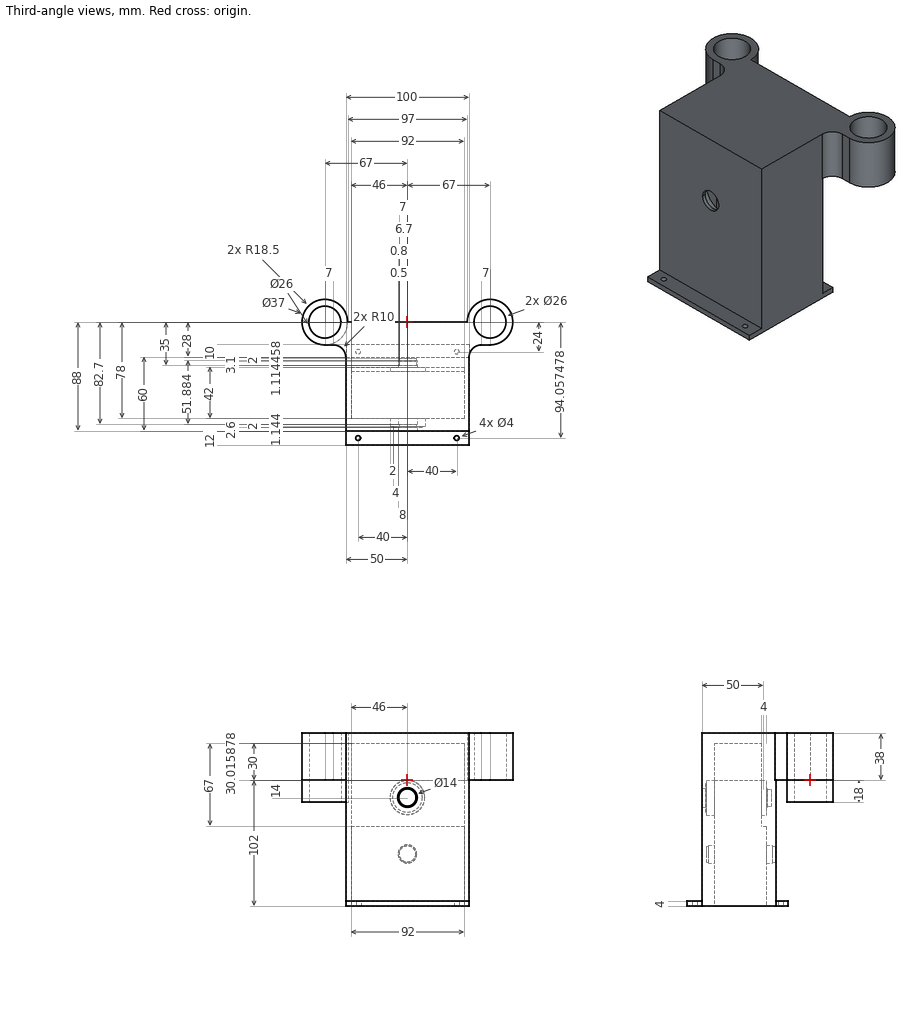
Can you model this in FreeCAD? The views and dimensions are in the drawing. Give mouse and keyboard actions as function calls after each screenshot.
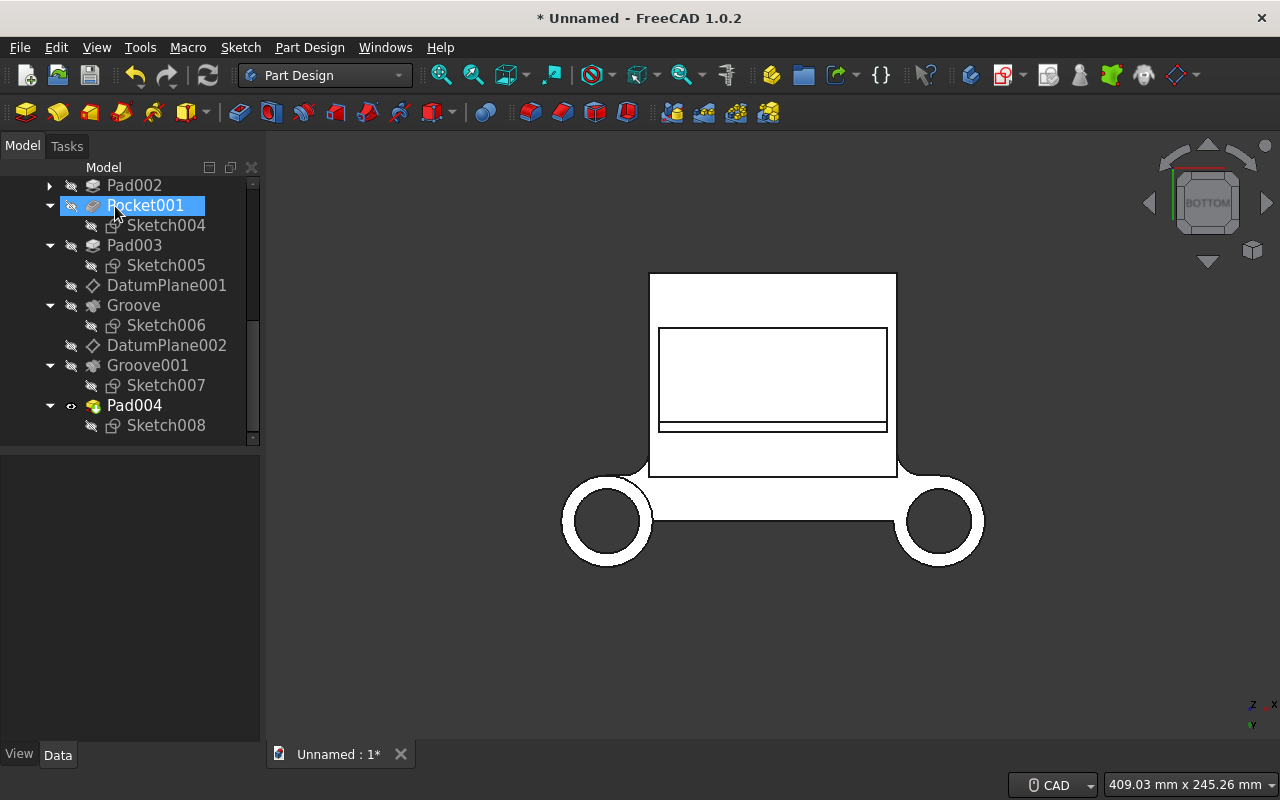
click(879, 461)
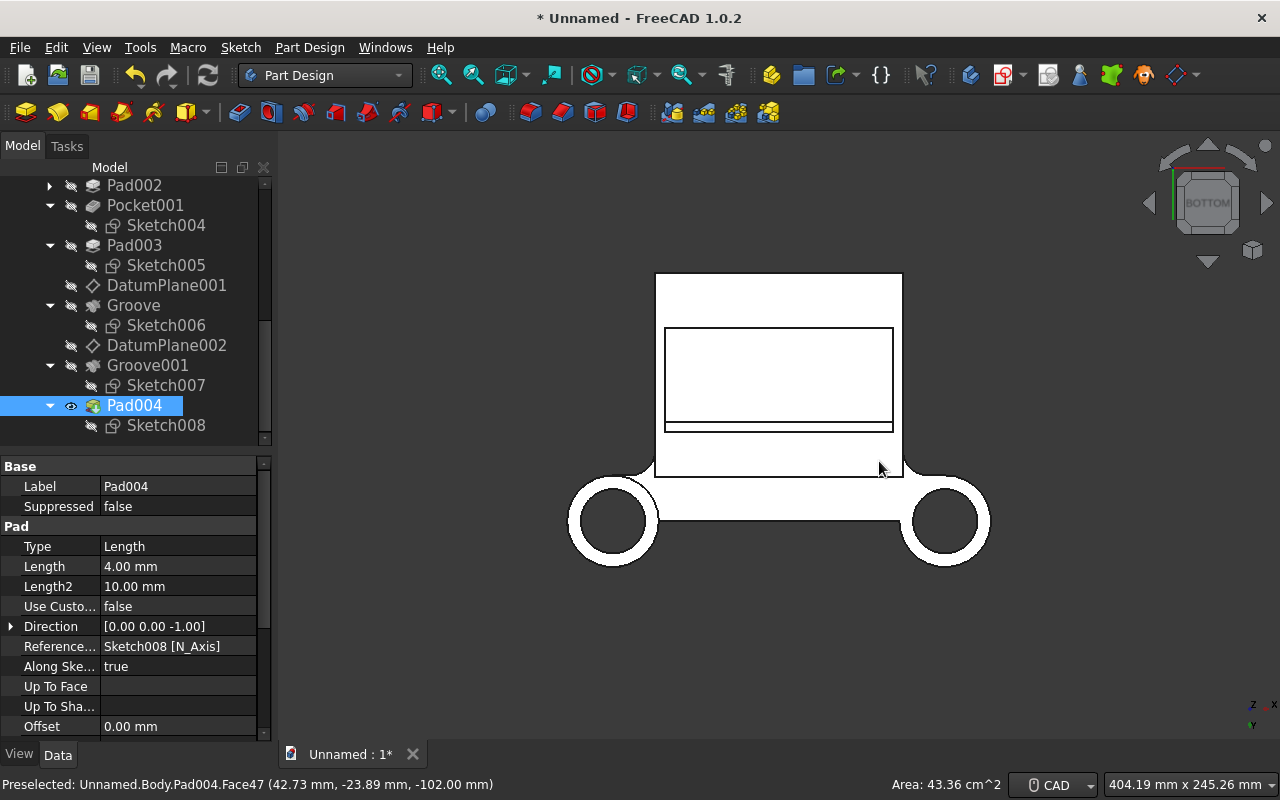
click(1004, 76)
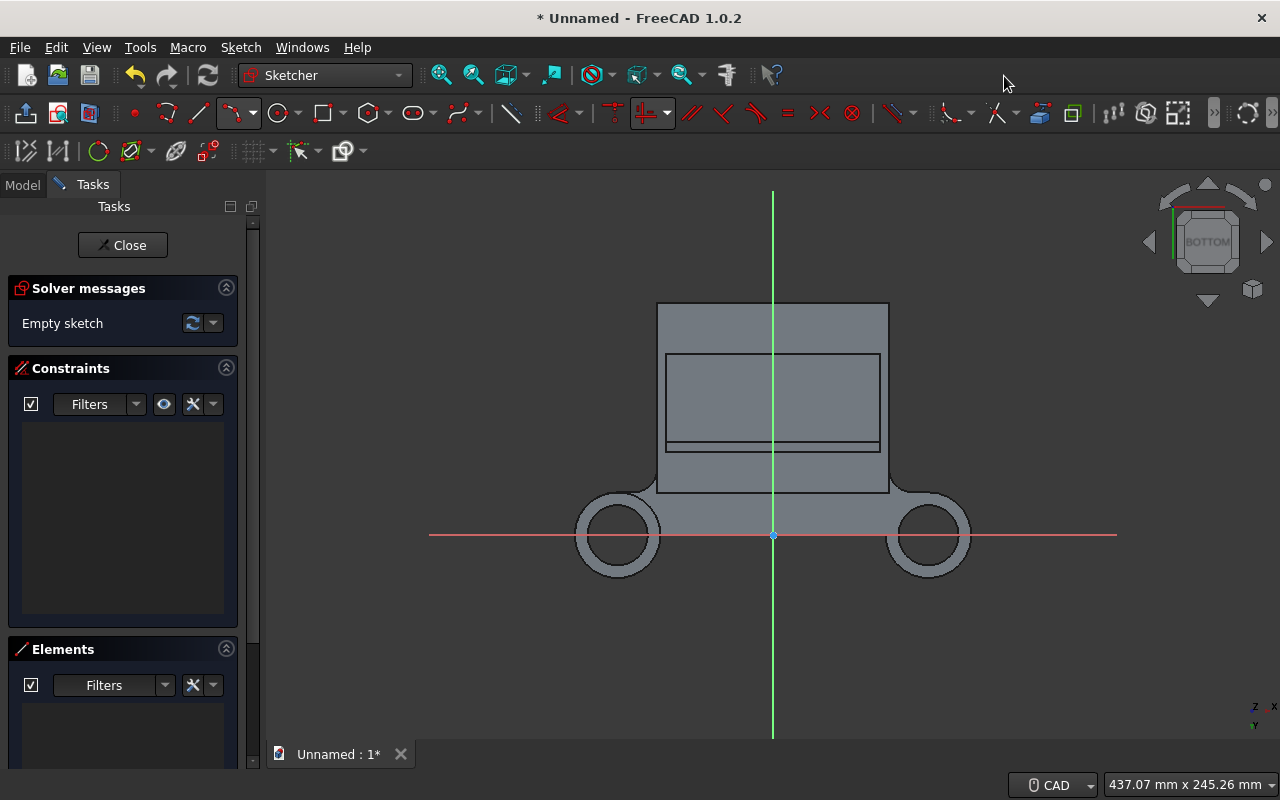
scroll(912, 361, up, 2)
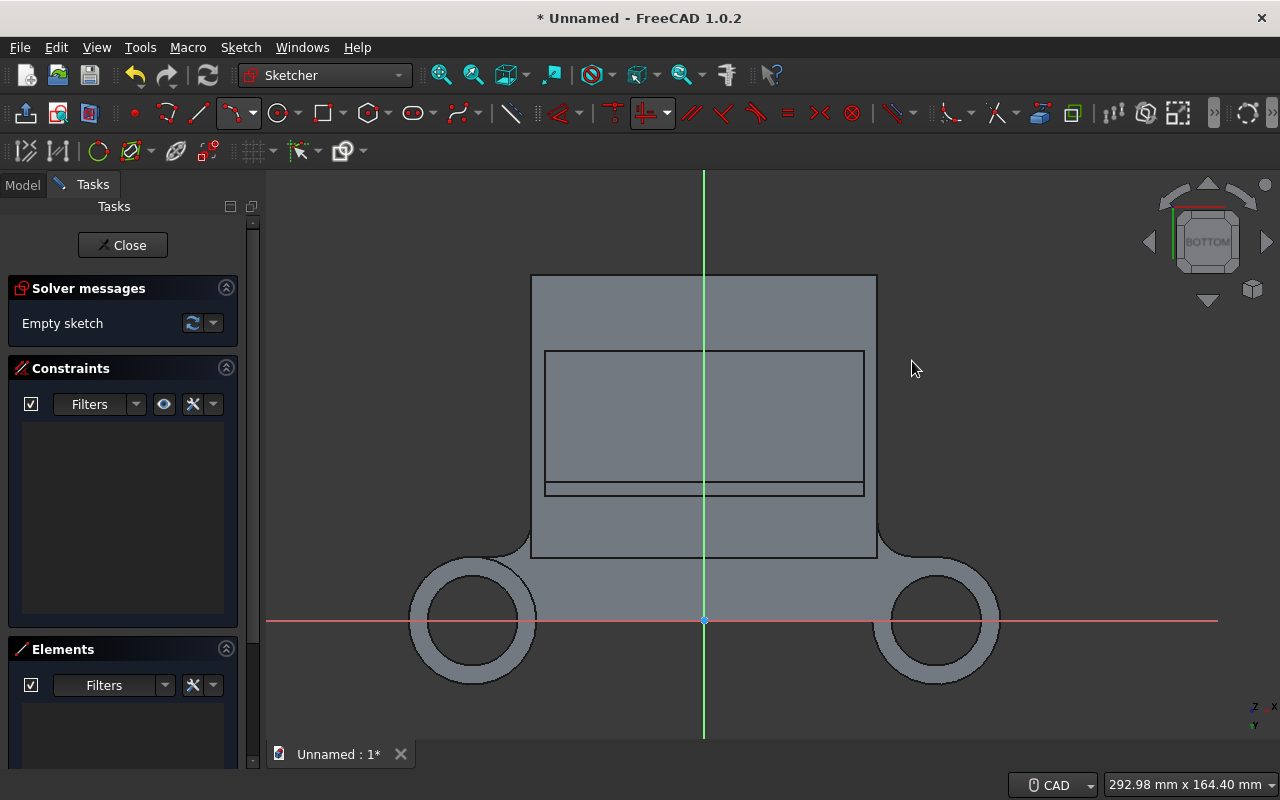
key(g)
key(c)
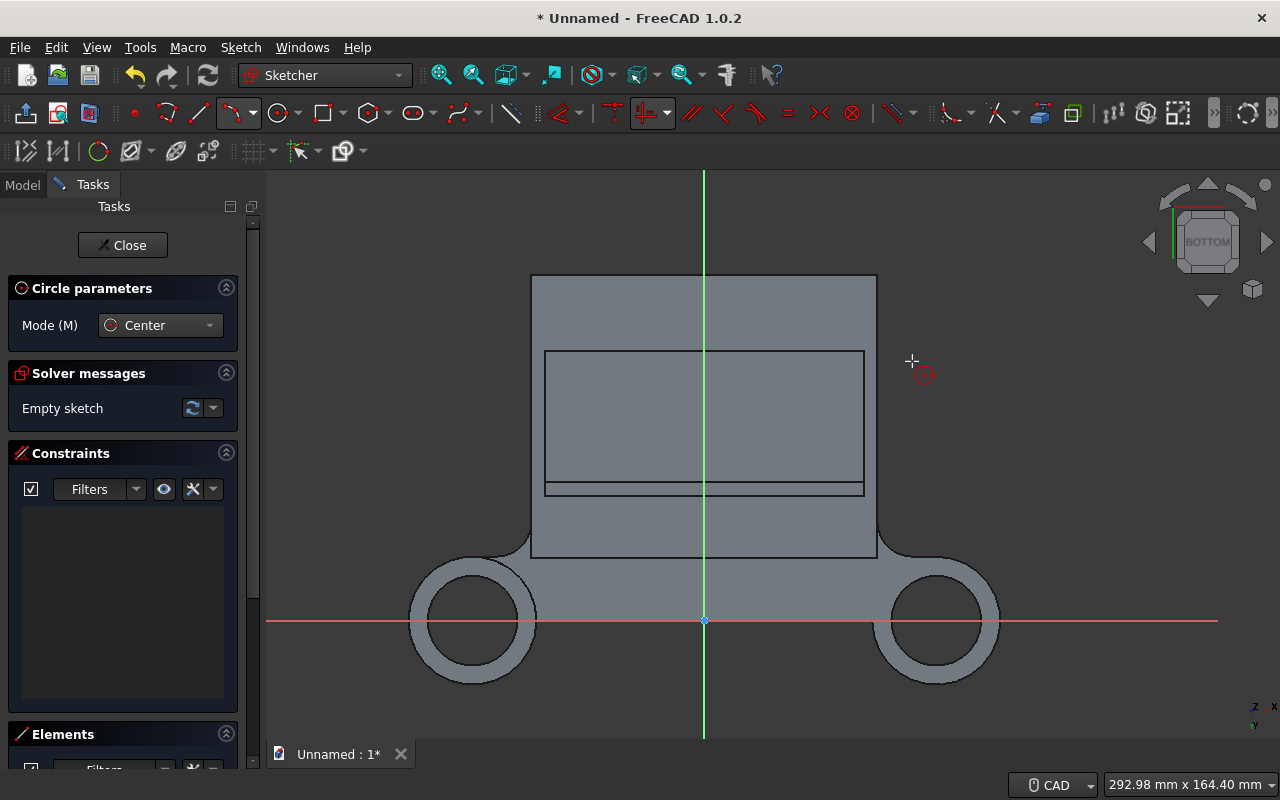
scroll(843, 295, up, 6)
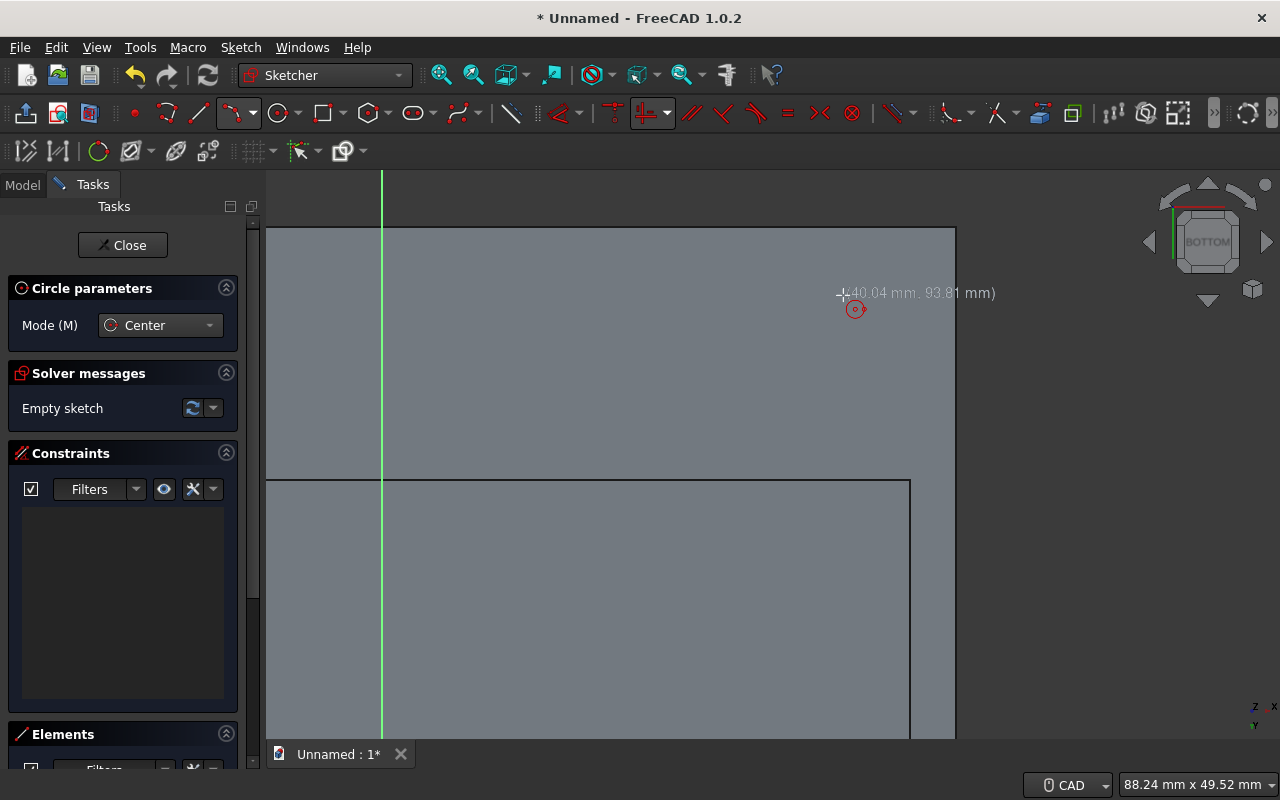
click(841, 295)
click(857, 279)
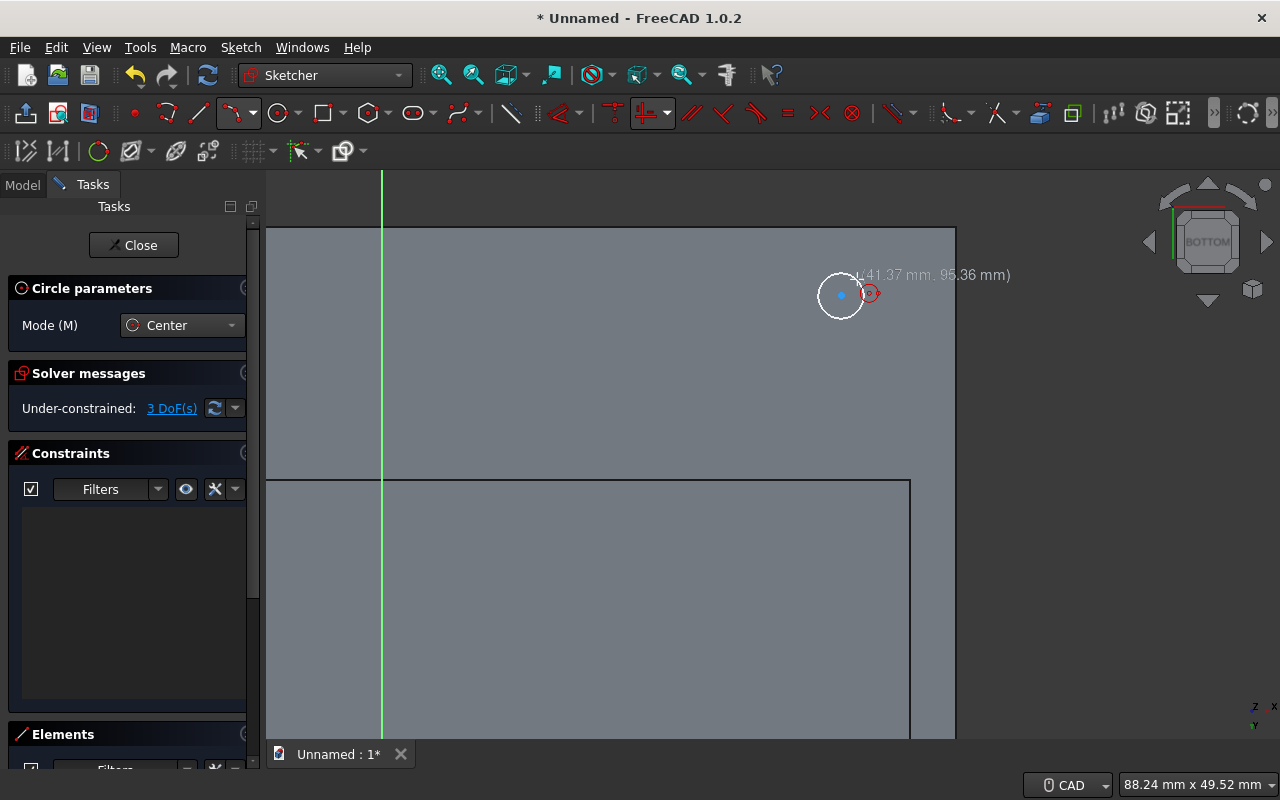
scroll(844, 295, down, 6)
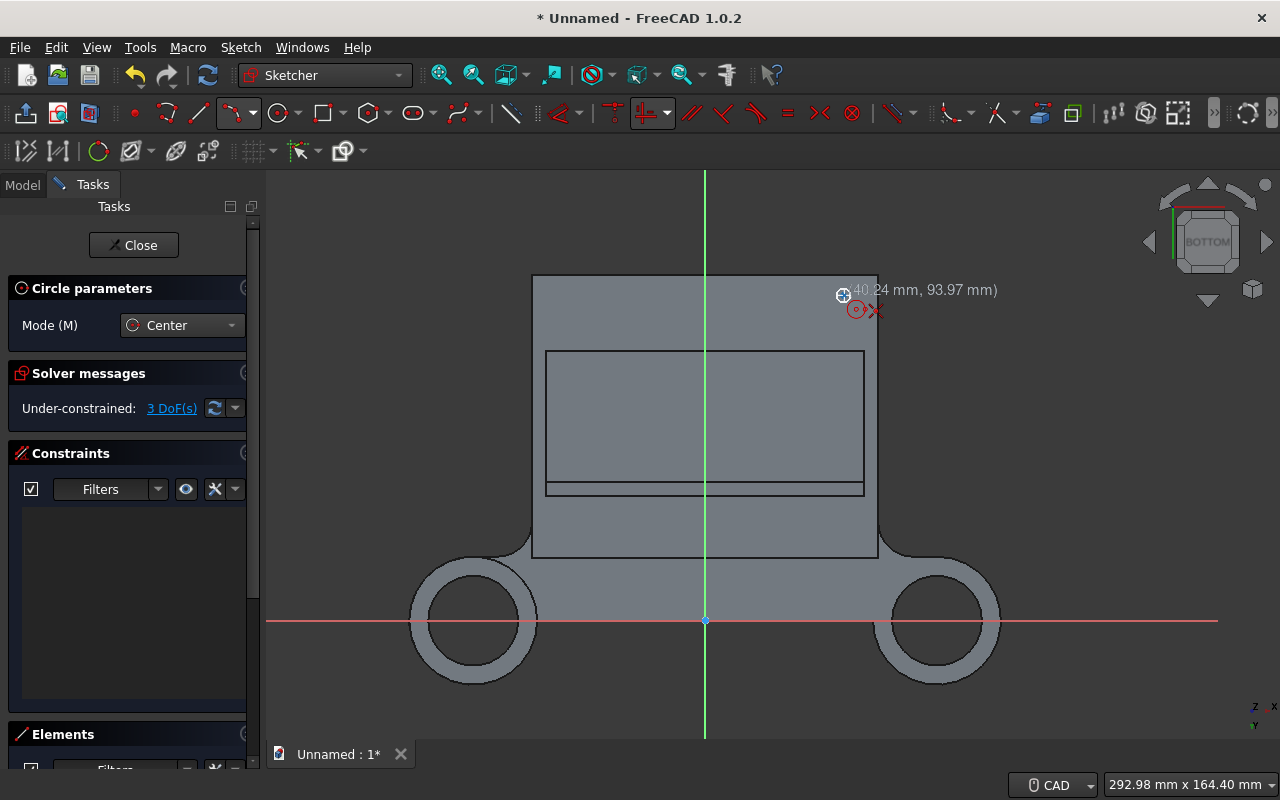
scroll(844, 538, up, 6)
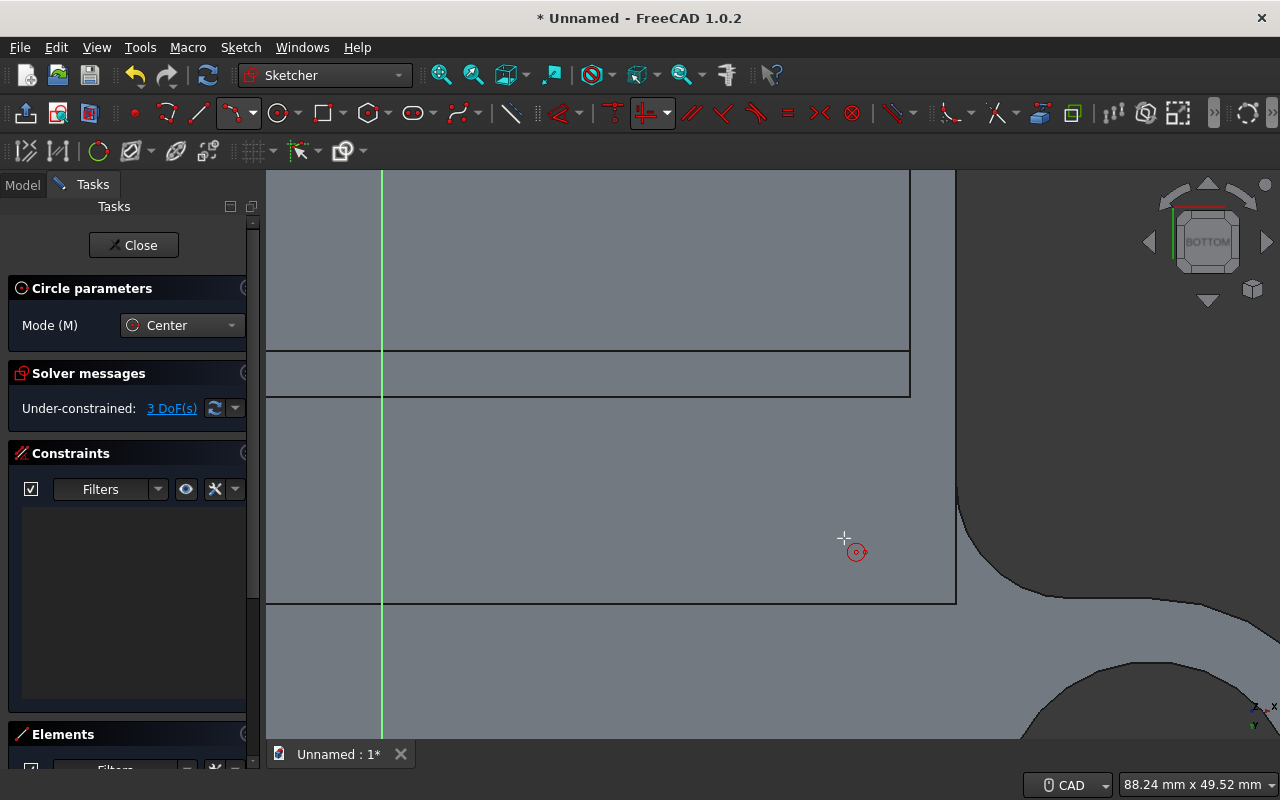
click(841, 535)
click(857, 519)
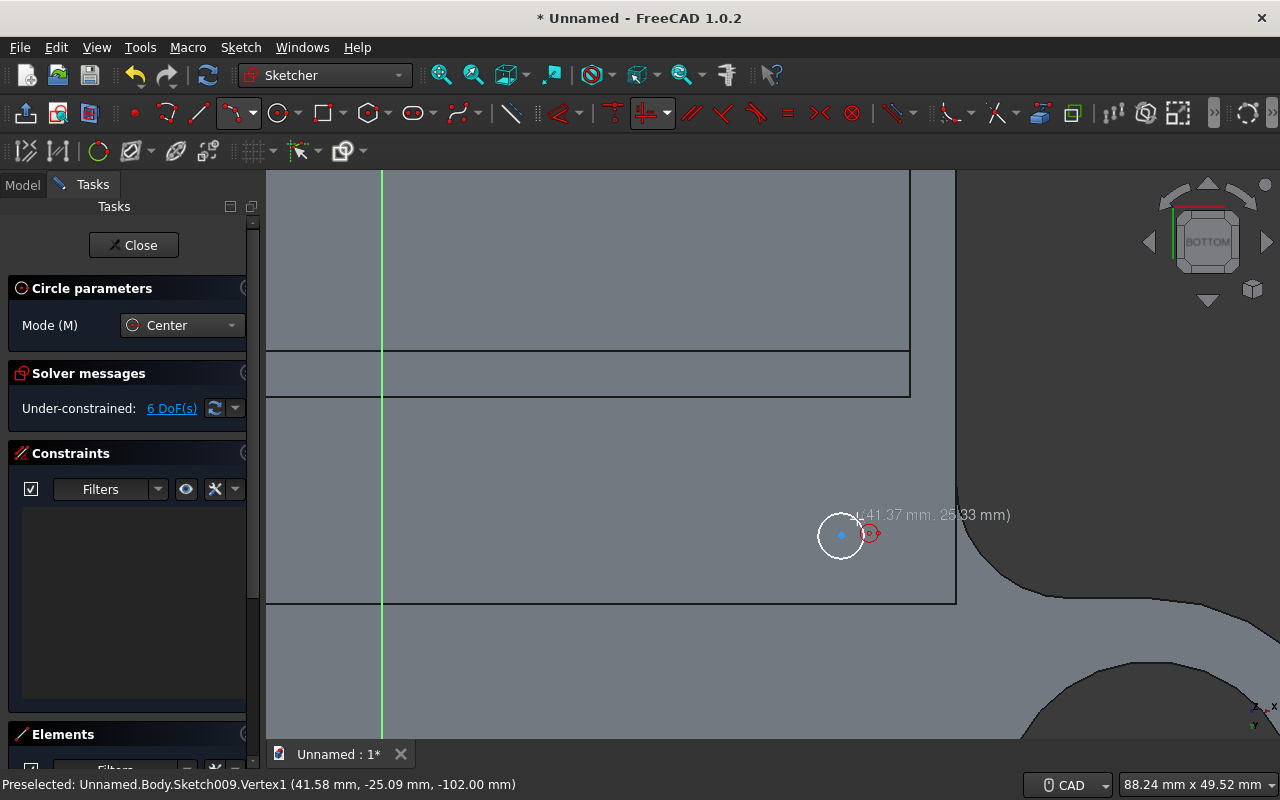
scroll(844, 539, down, 6)